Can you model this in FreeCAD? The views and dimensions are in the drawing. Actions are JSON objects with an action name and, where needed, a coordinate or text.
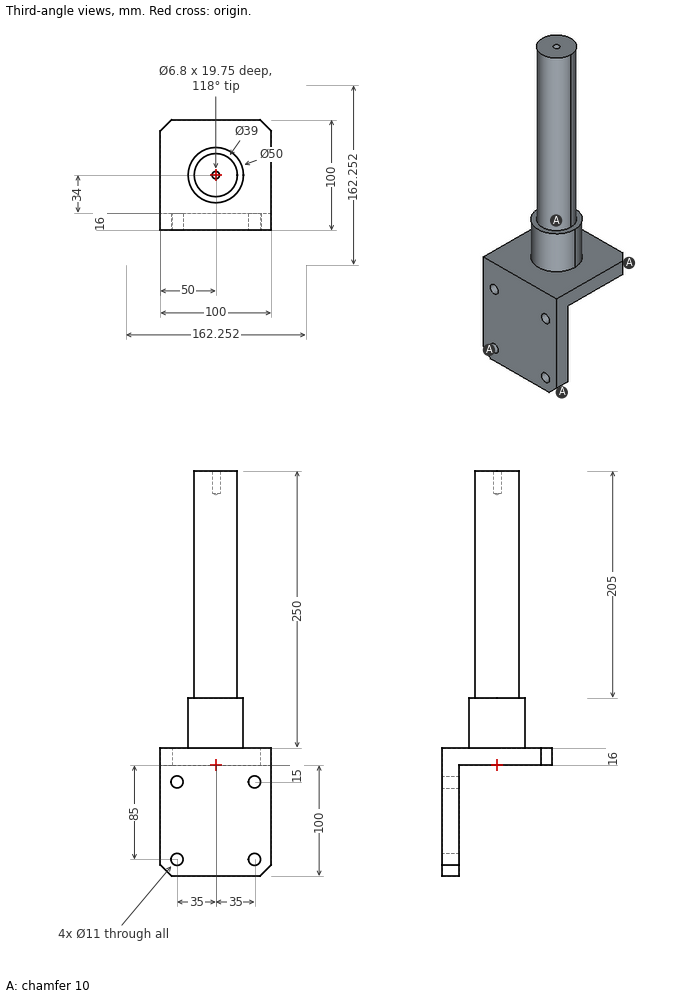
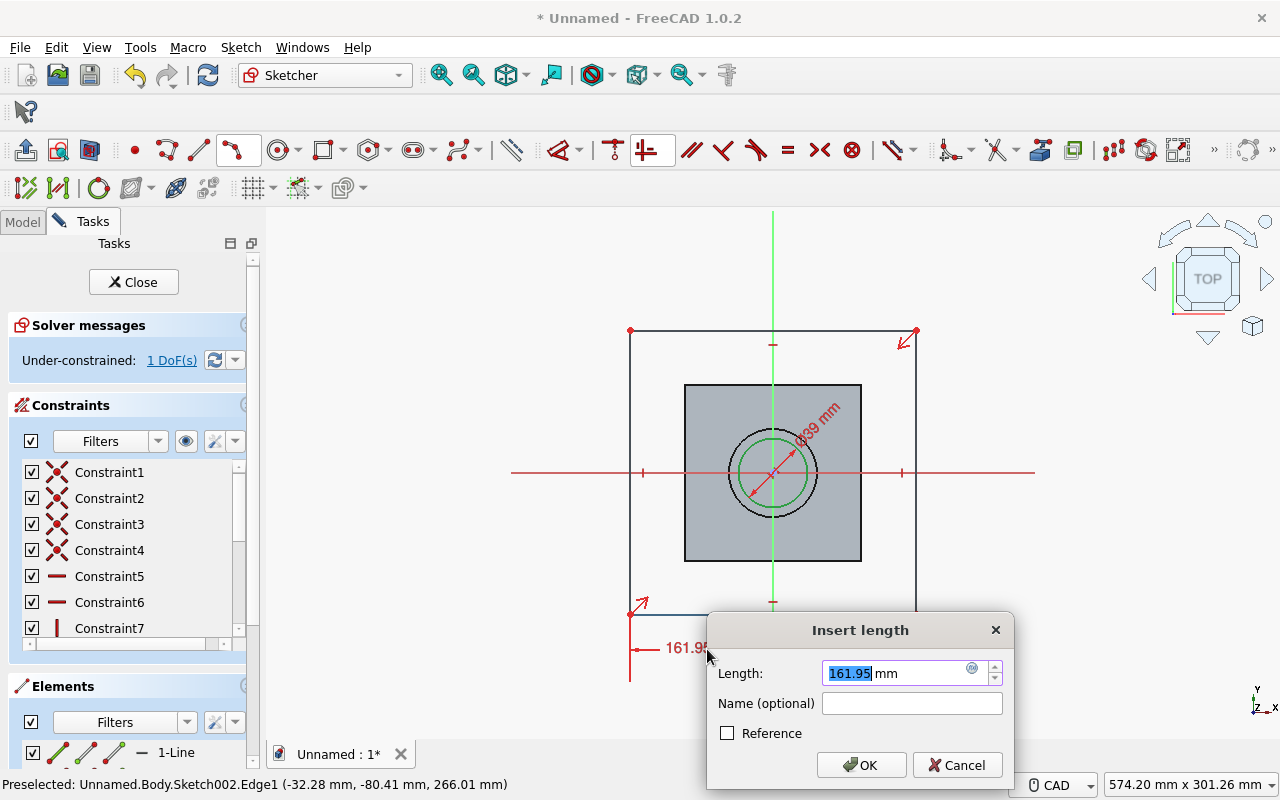
{"action": "type", "text": "162.252"}
{"action": "key", "text": "Return"}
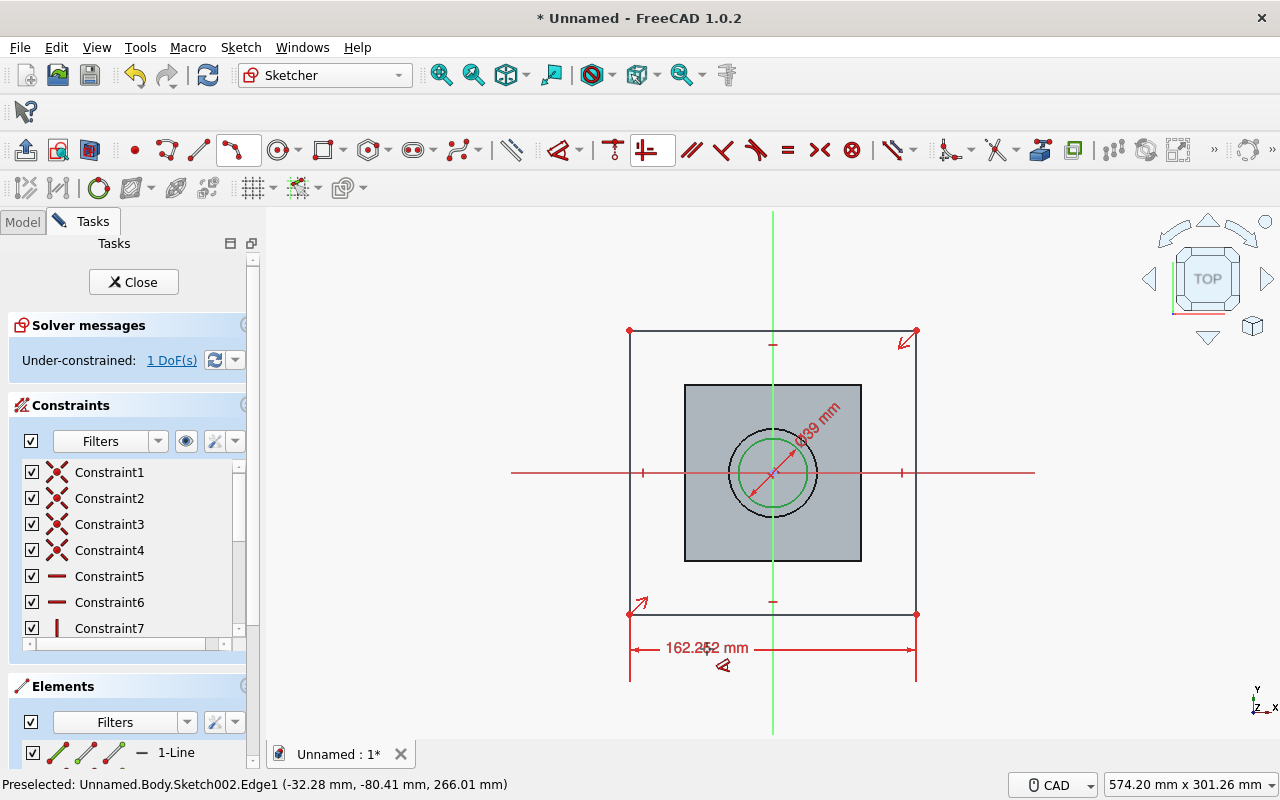
{"action": "left_click", "coordinate": [916, 530]}
{"action": "left_click", "coordinate": [950, 408]}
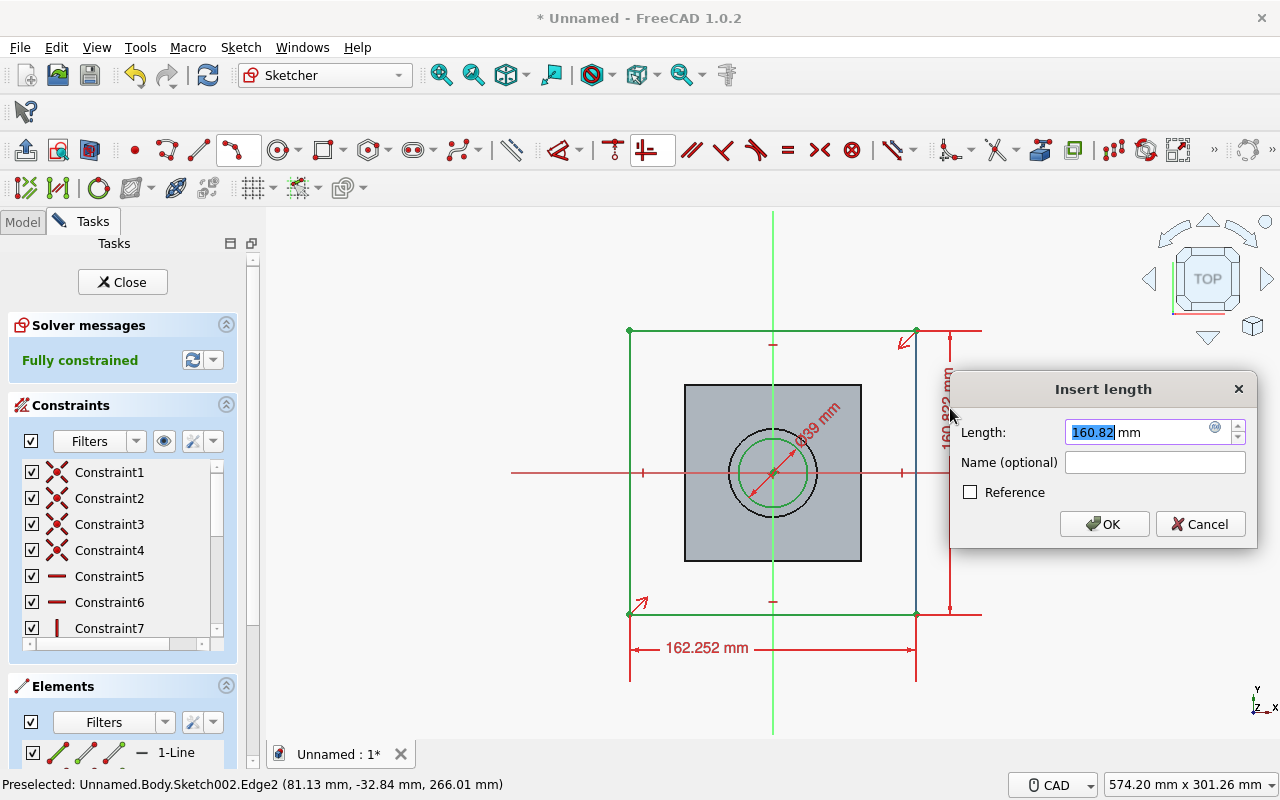
{"action": "type", "text": "162.252"}
{"action": "key", "text": "Return"}
{"action": "key", "text": "Escape"}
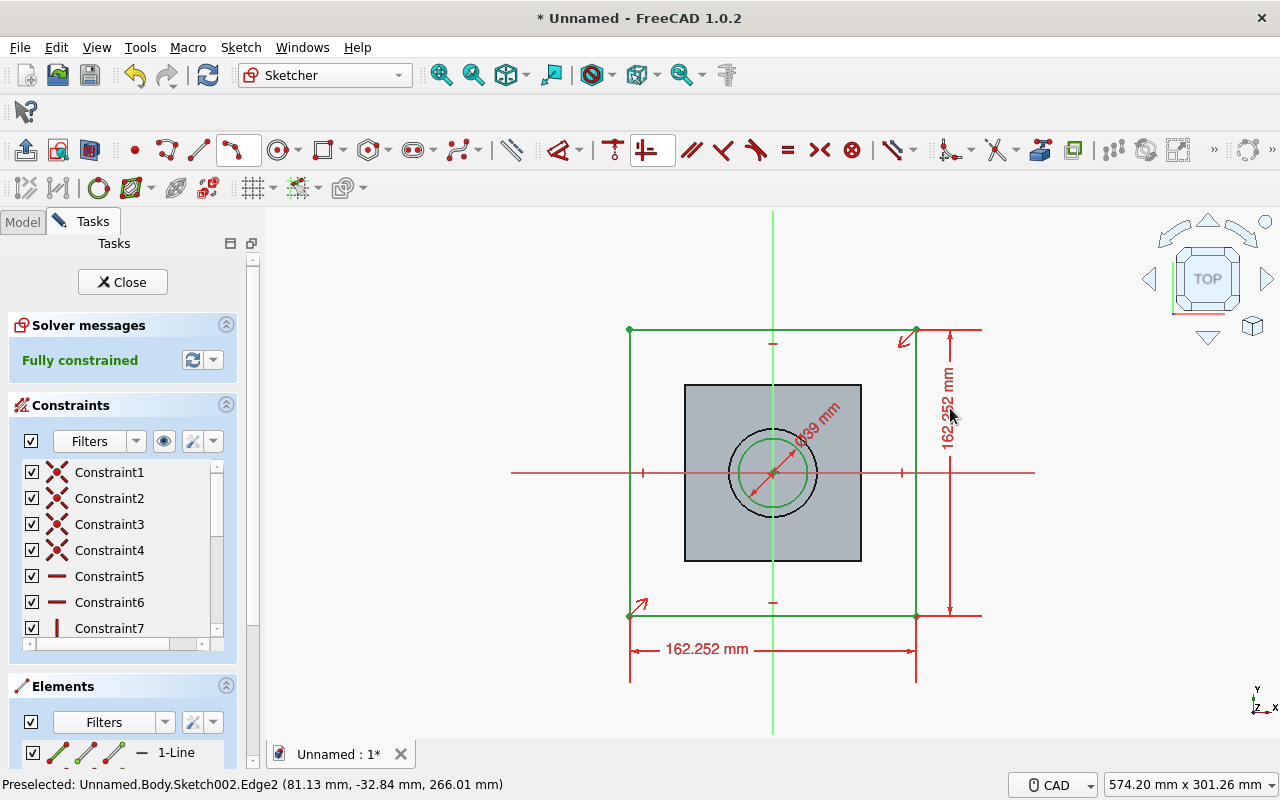
{"action": "left_click", "coordinate": [123, 282]}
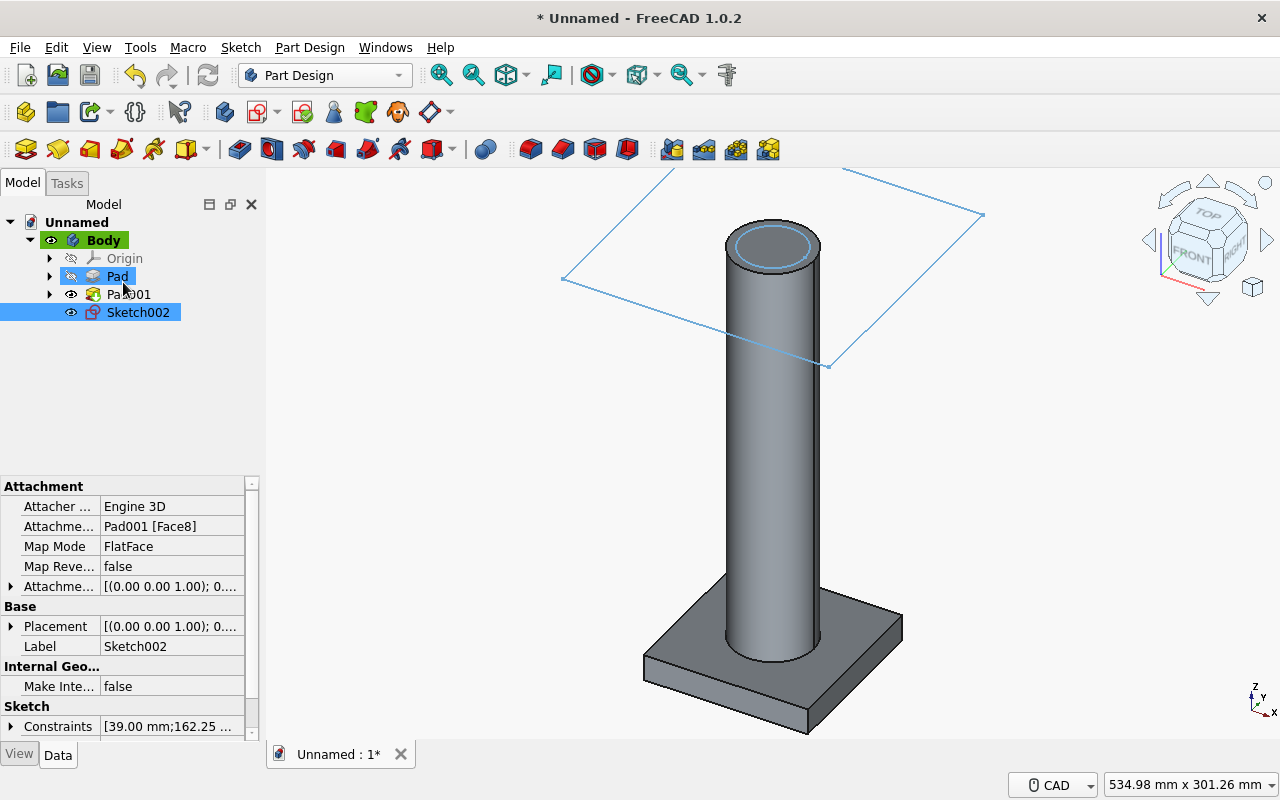
{"action": "left_click", "coordinate": [240, 150]}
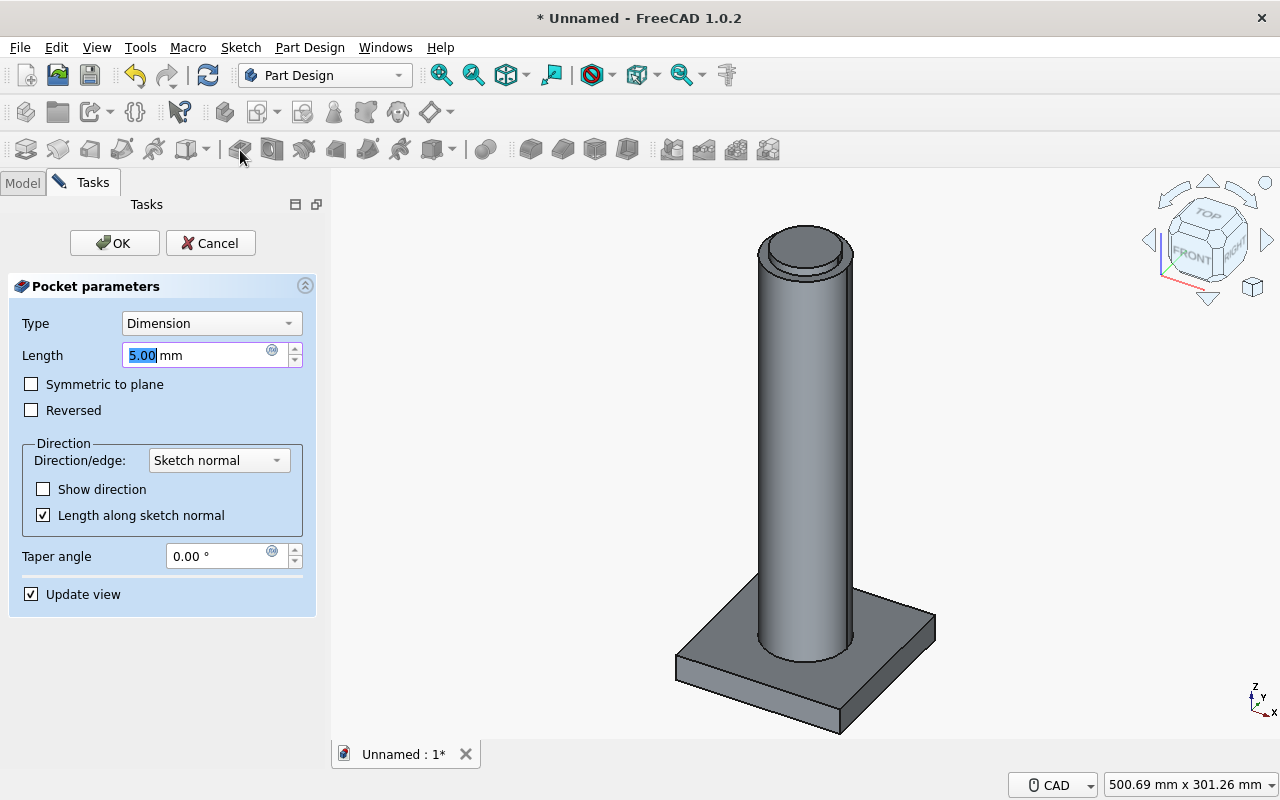
{"action": "type", "text": "205"}
{"action": "key", "text": "Tab"}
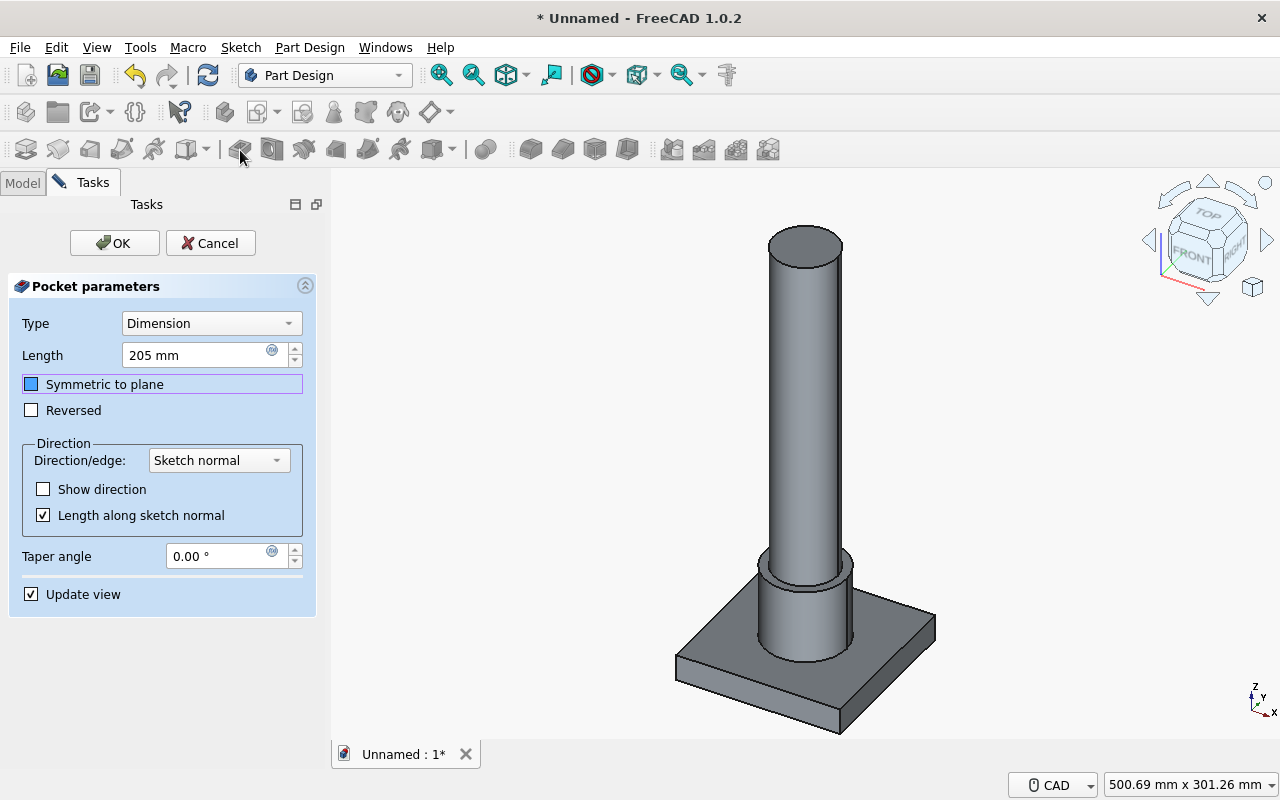
{"action": "left_click", "coordinate": [115, 243]}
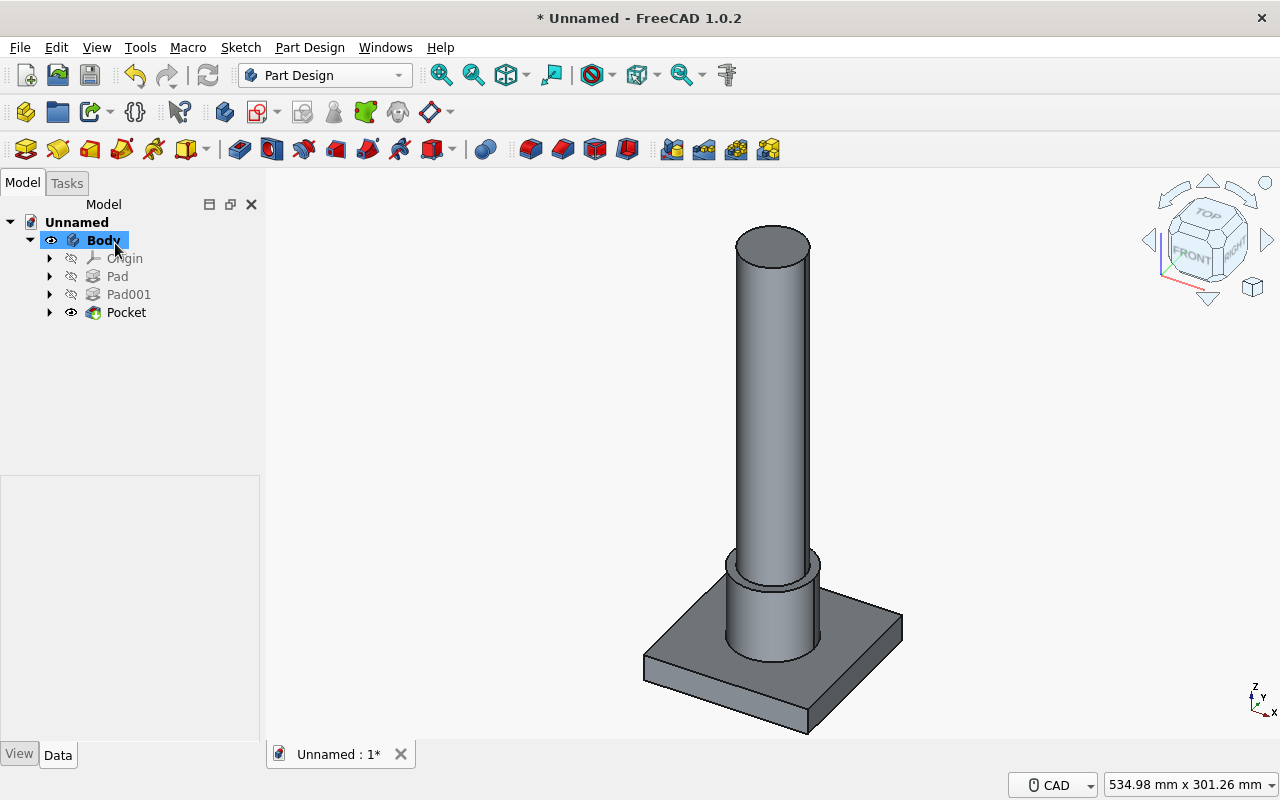
{"action": "left_click", "coordinate": [258, 112]}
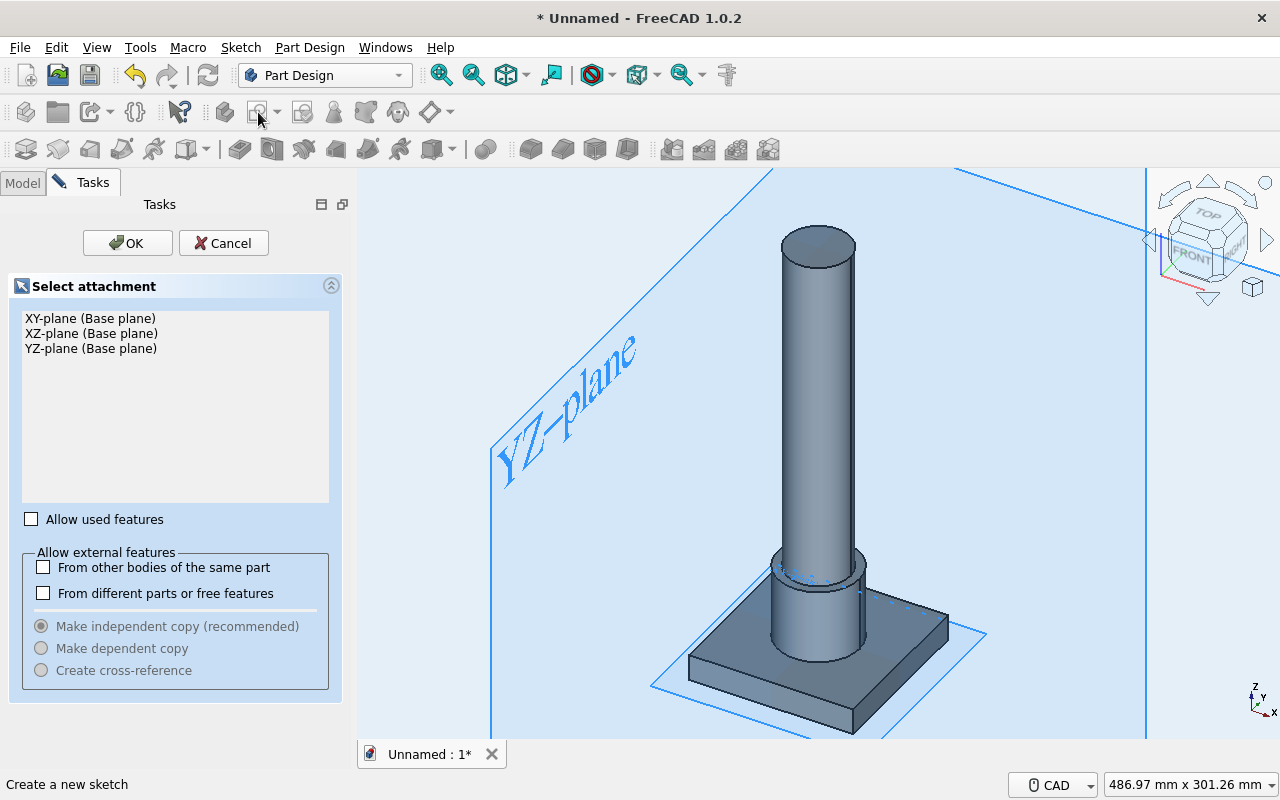
{"action": "left_click", "coordinate": [82, 318]}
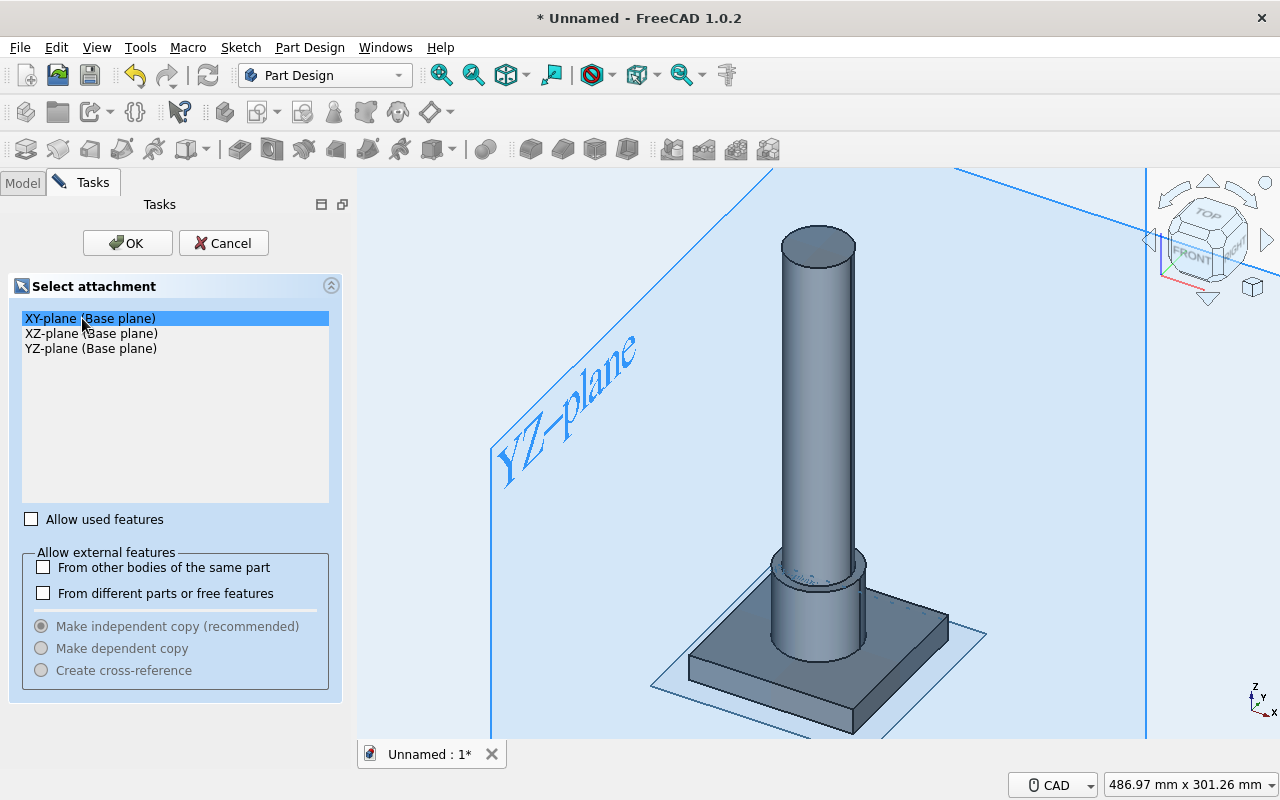
{"action": "left_click", "coordinate": [128, 243]}